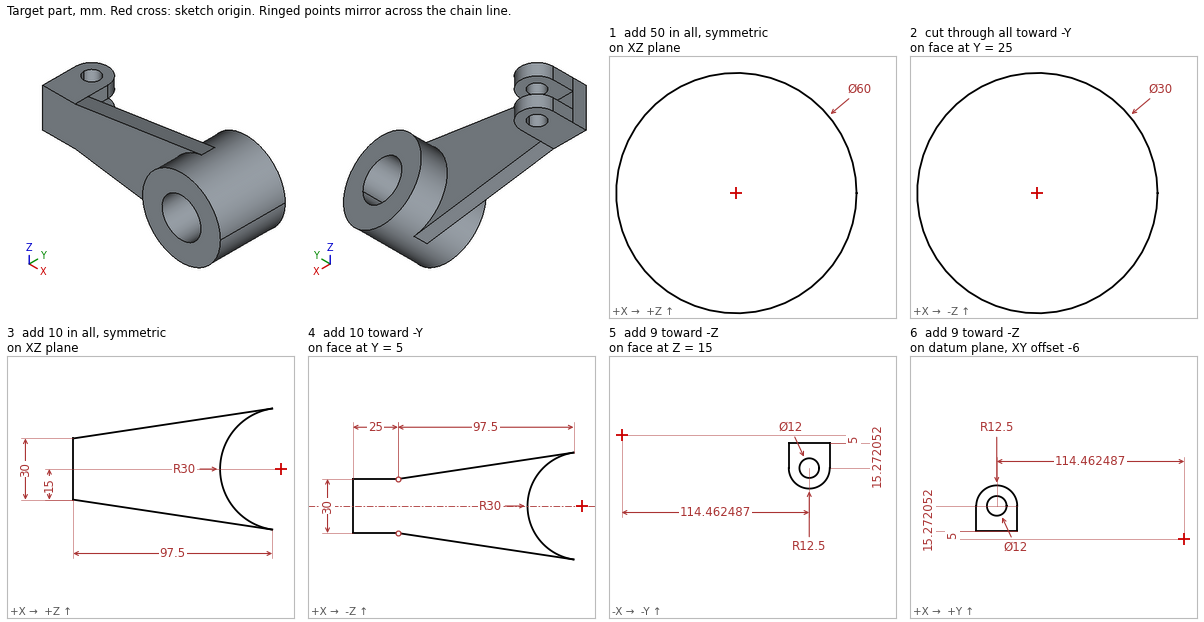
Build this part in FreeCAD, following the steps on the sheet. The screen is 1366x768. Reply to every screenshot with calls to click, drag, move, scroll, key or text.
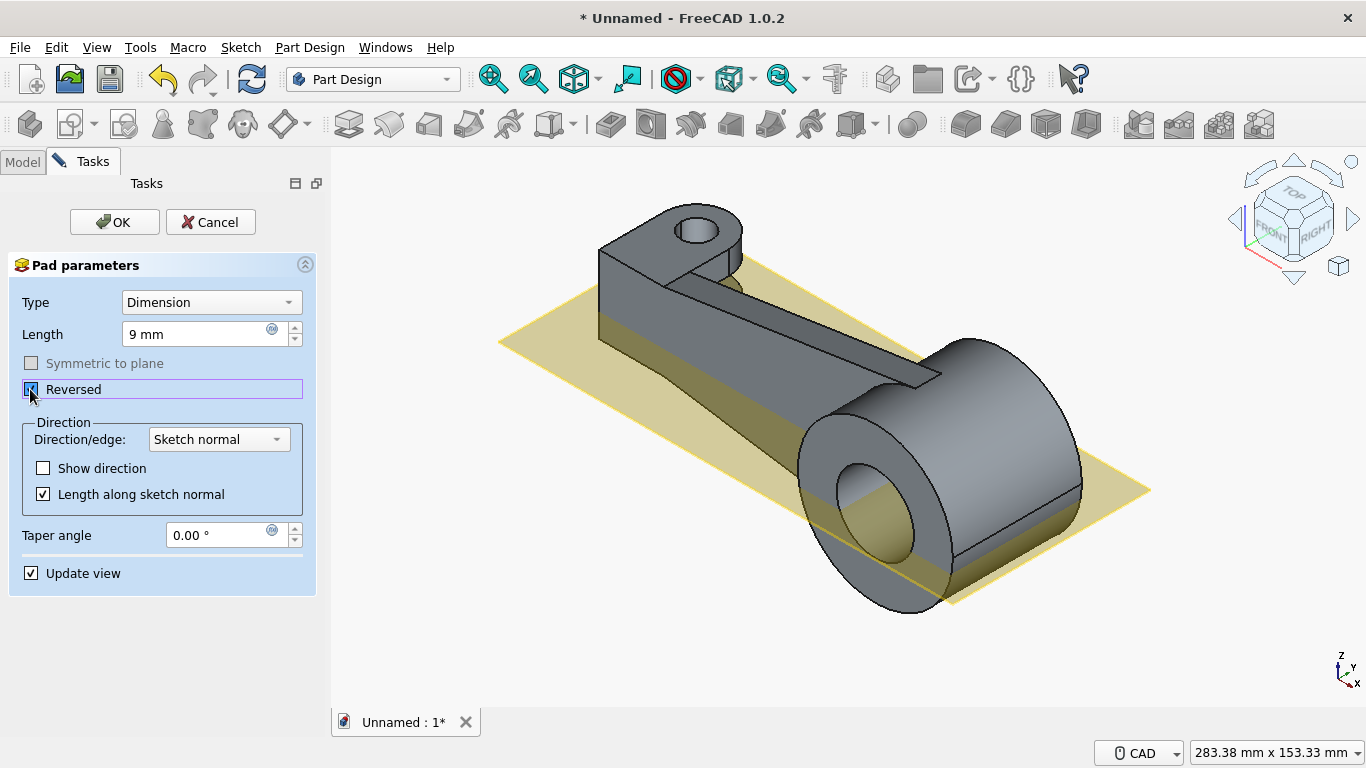
click(115, 222)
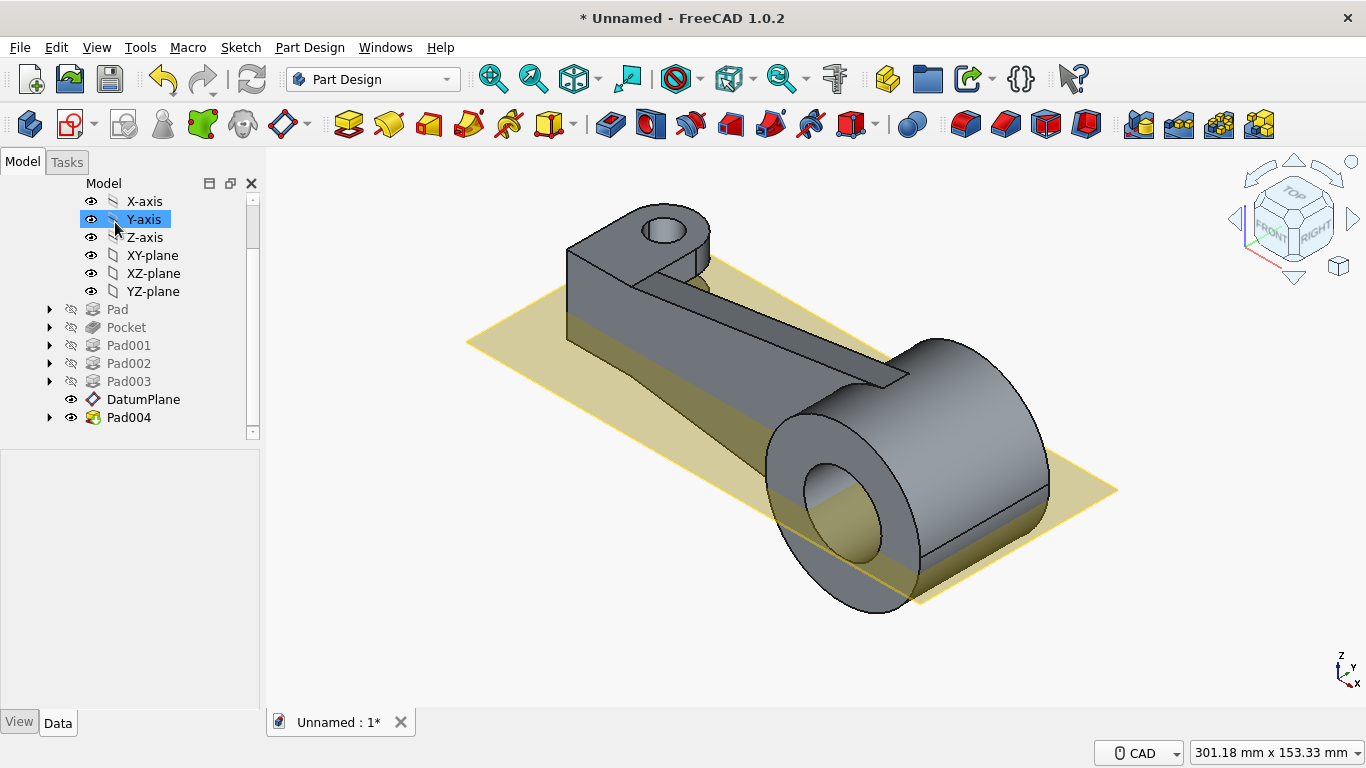
click(116, 399)
key(space)